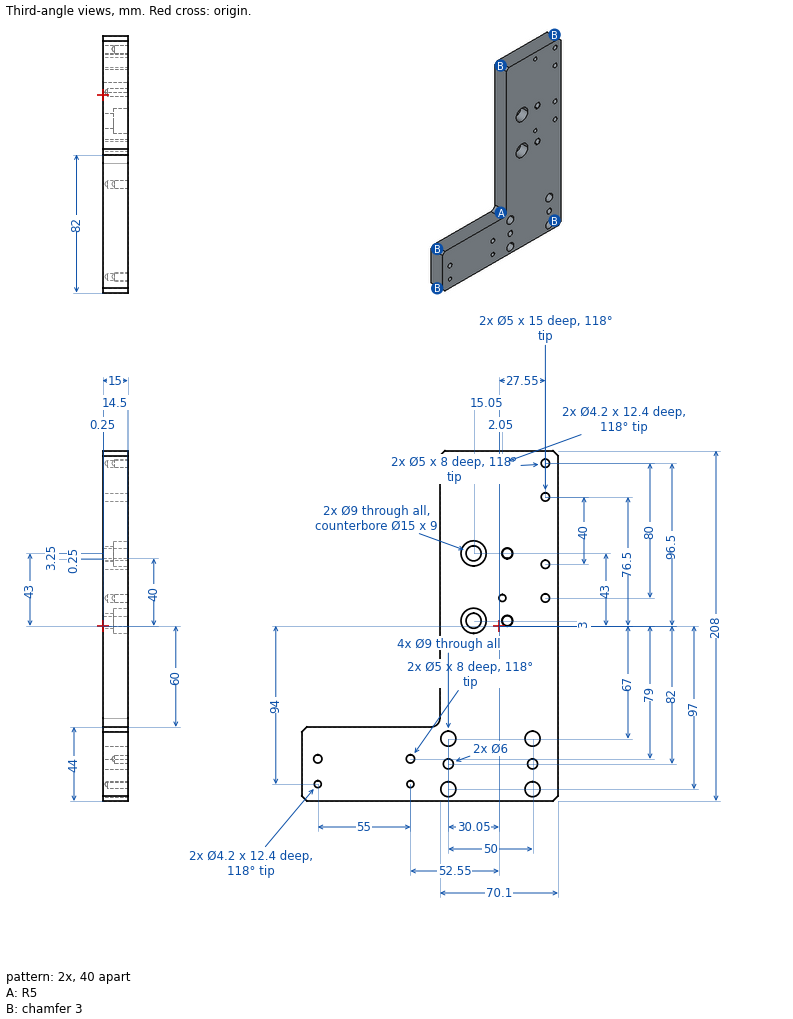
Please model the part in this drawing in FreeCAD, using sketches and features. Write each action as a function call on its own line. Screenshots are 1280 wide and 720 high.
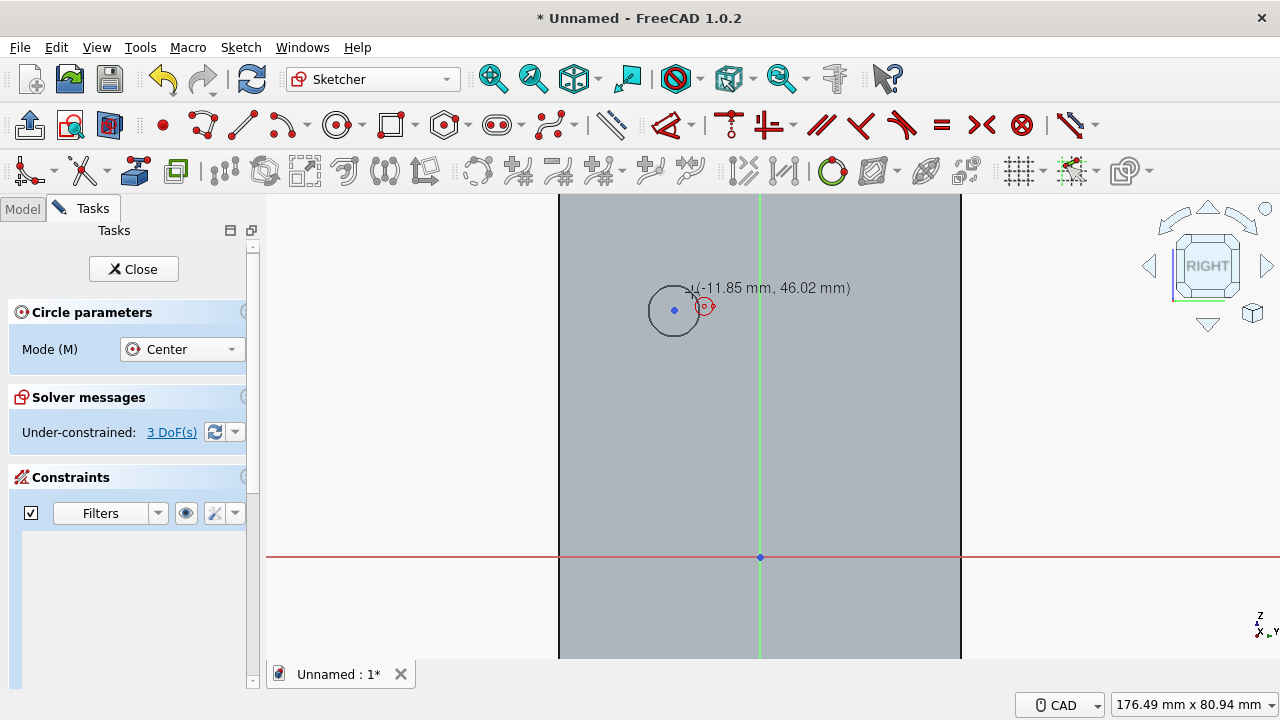
click(674, 540)
click(692, 522)
key(Escape)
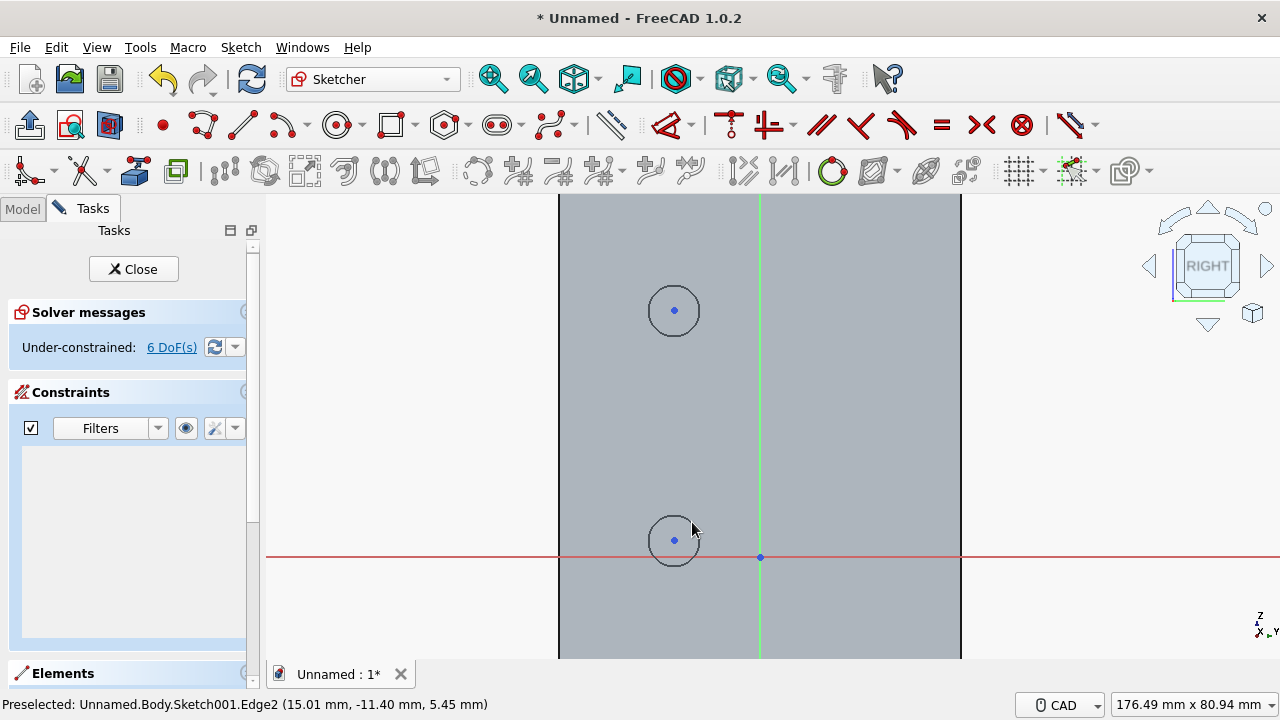
click(692, 293)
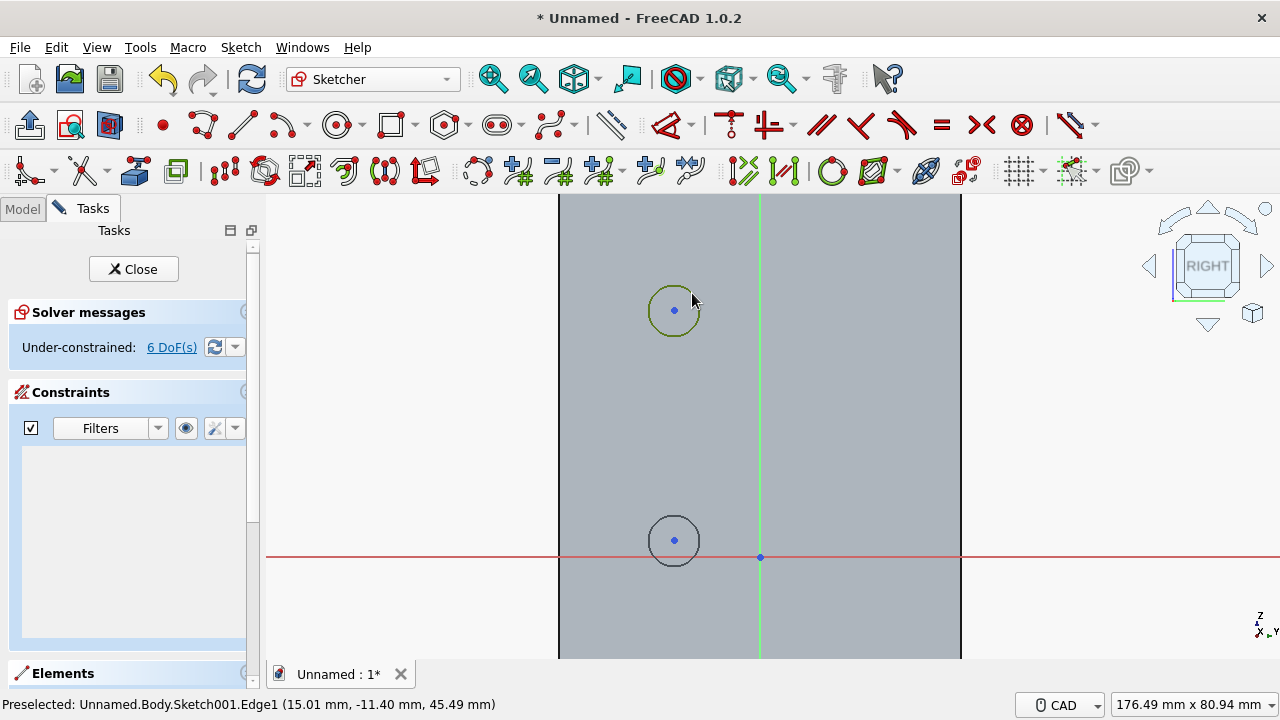
click(692, 523)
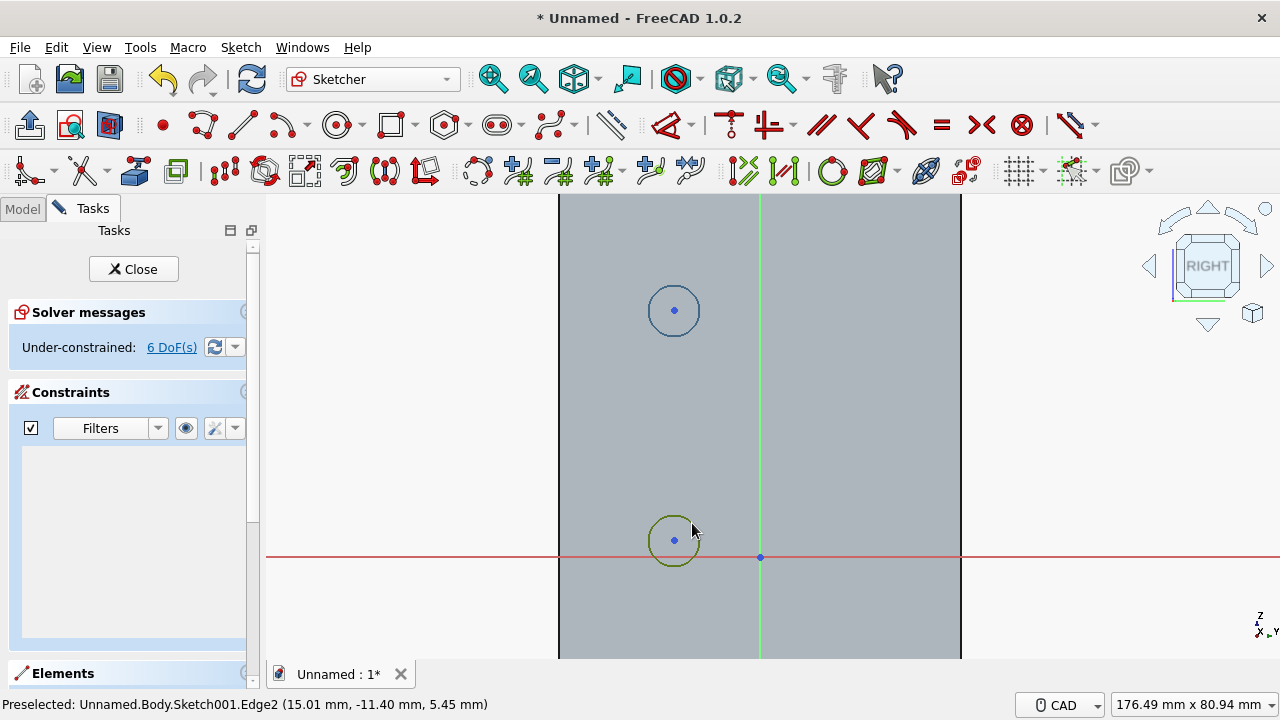
click(942, 126)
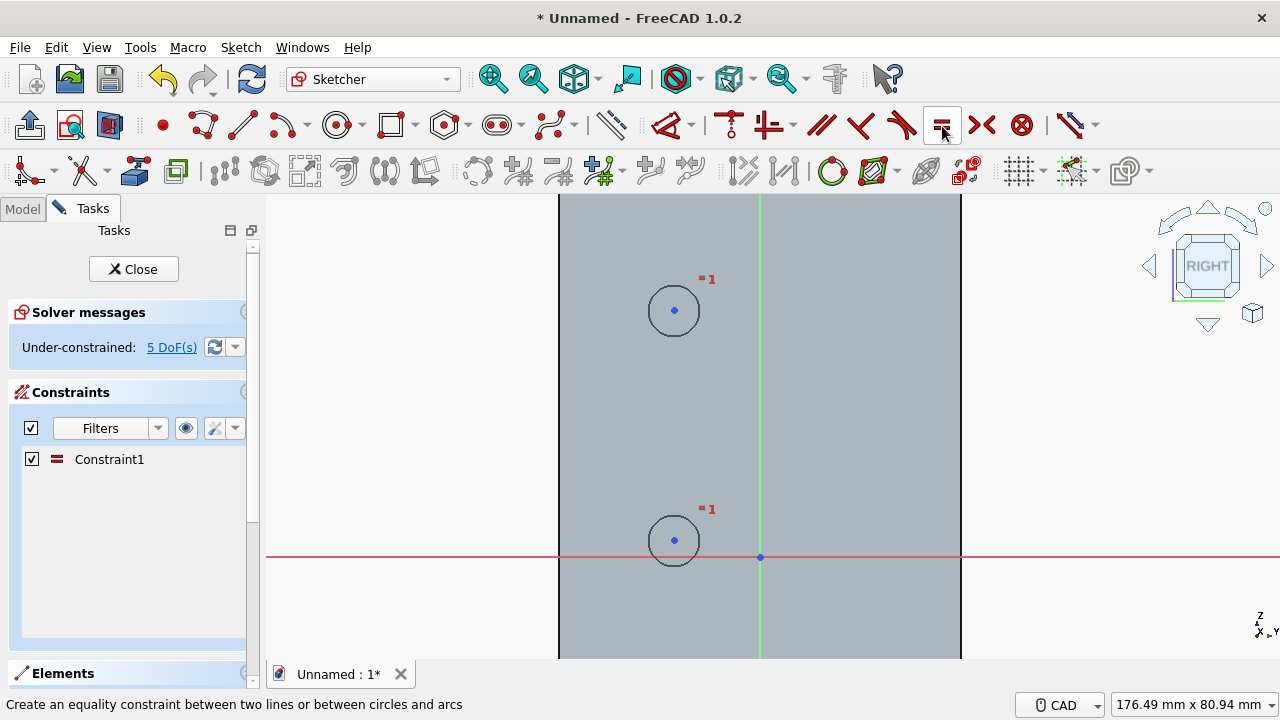
click(674, 311)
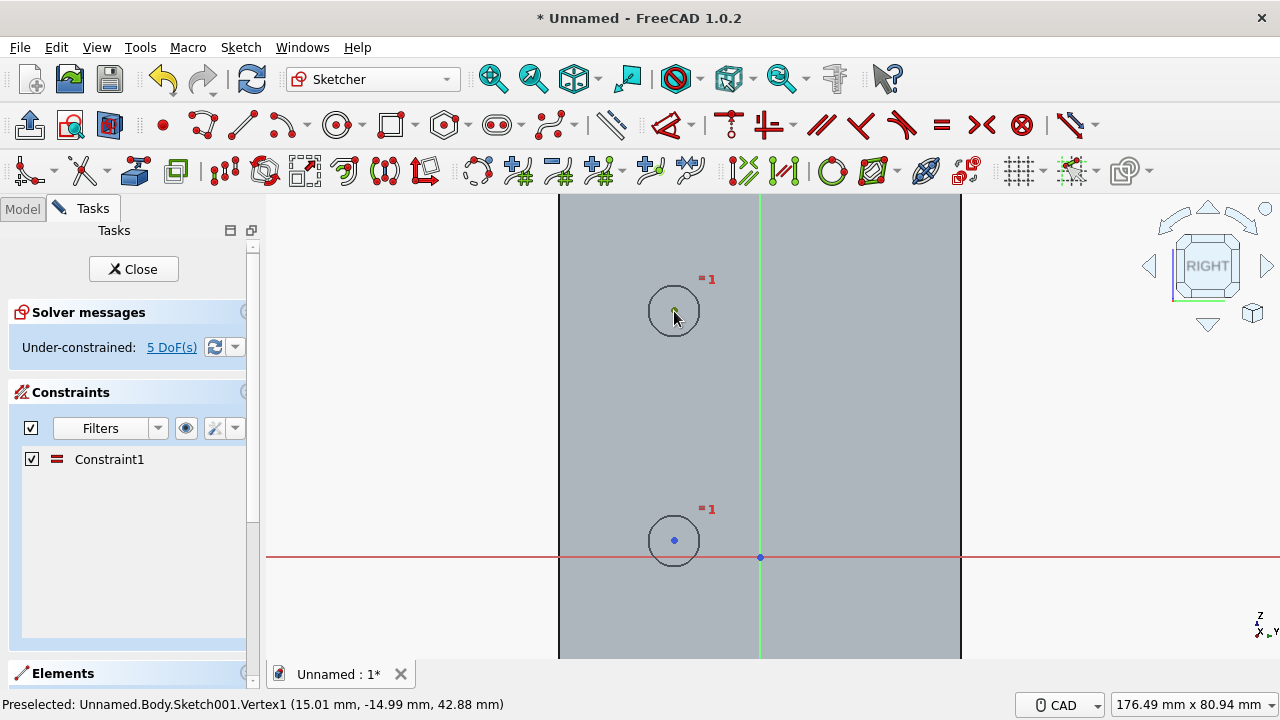
click(674, 541)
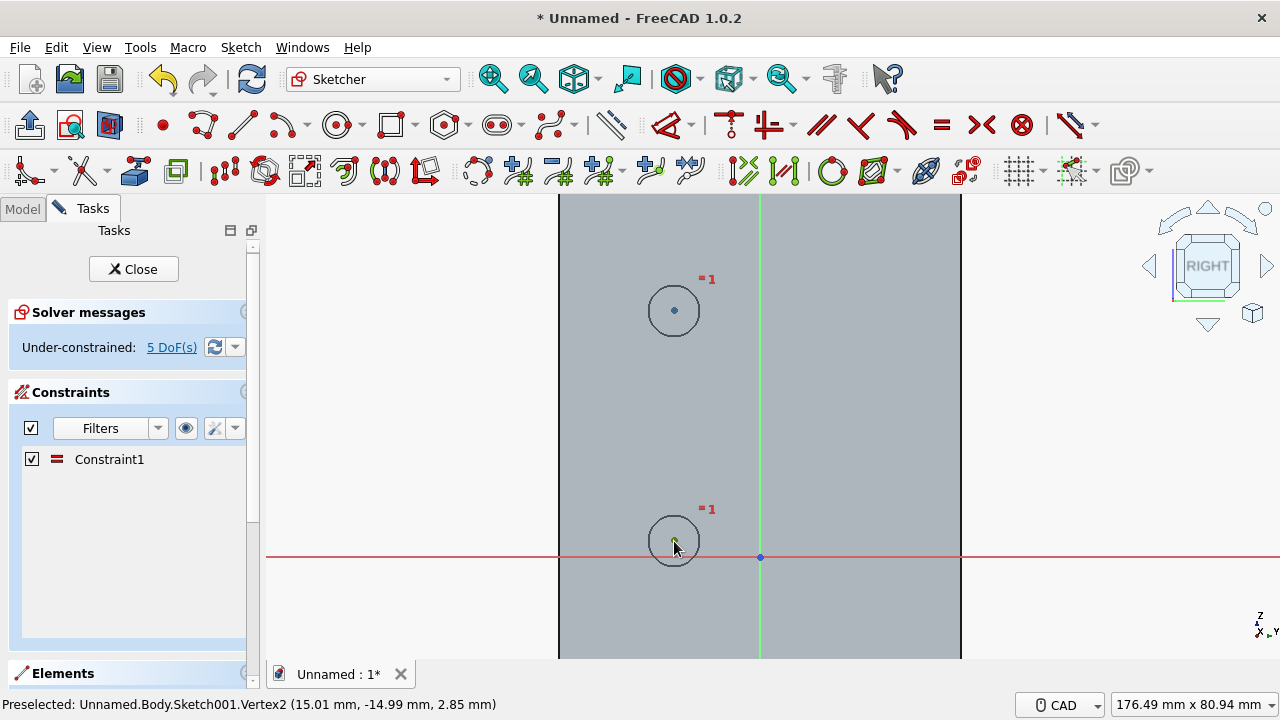
click(796, 126)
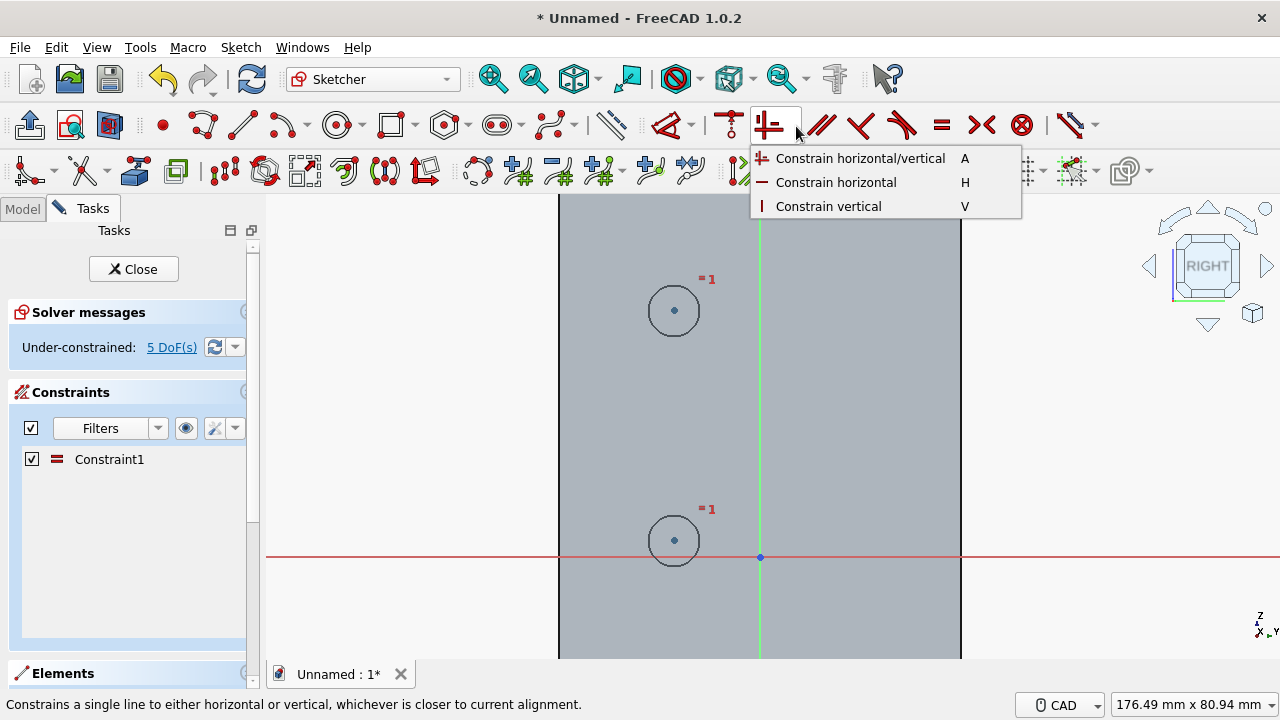
click(886, 206)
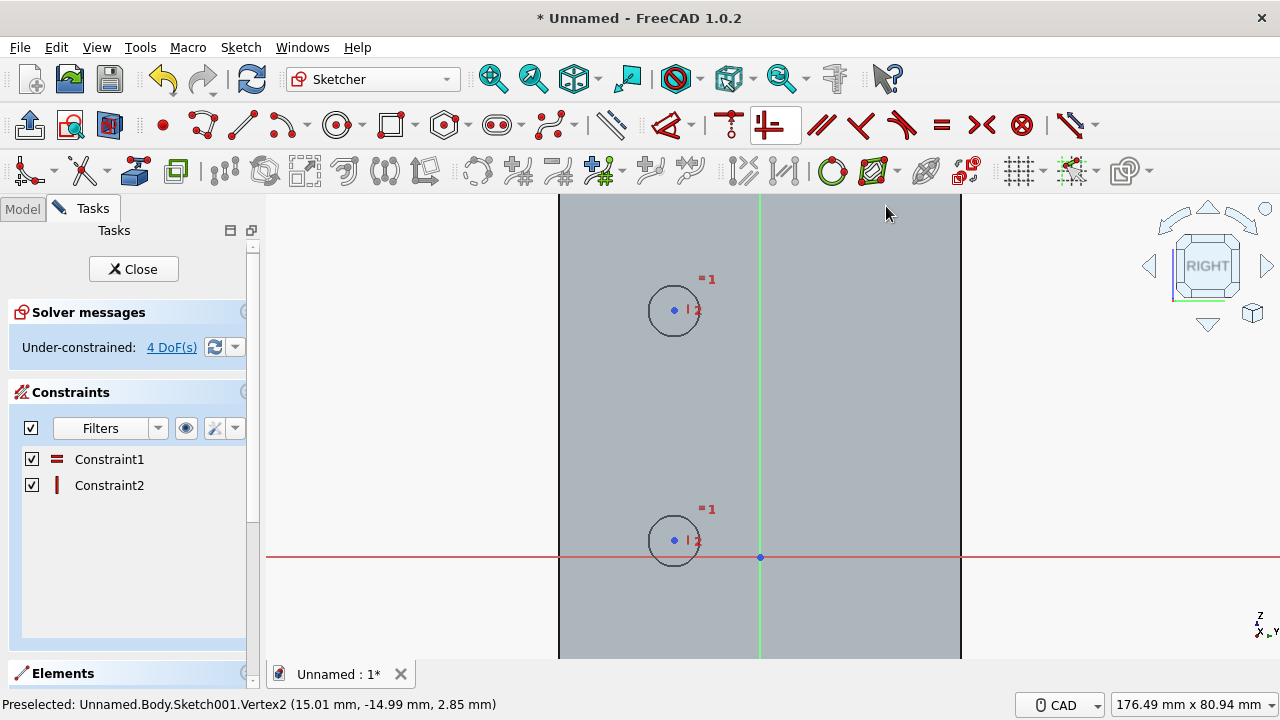
key(d)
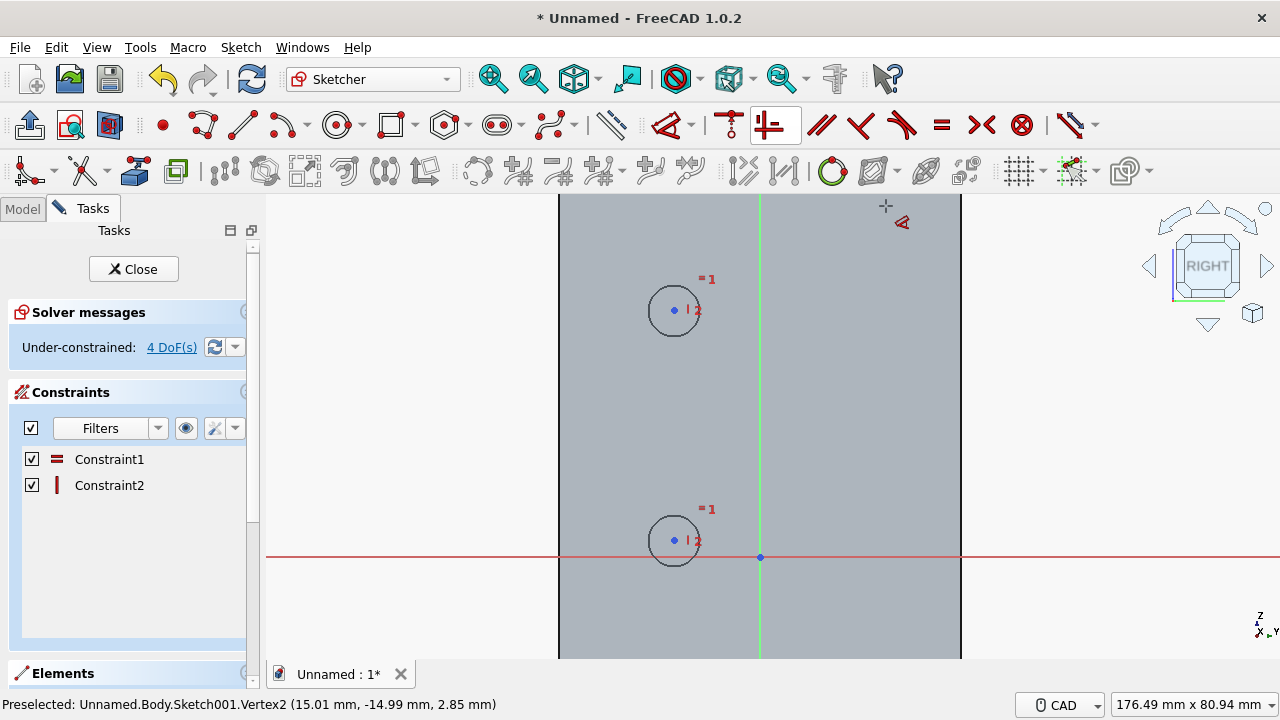
click(692, 293)
click(715, 270)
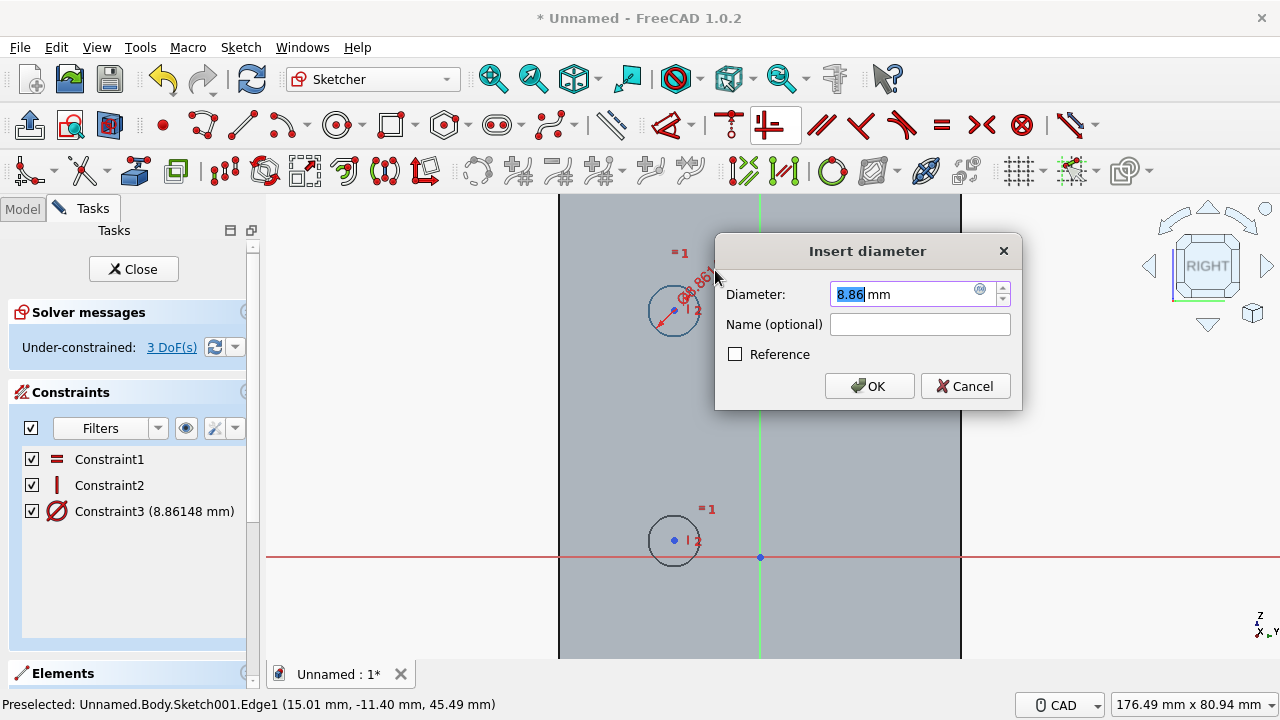
text(9)
key(Return)